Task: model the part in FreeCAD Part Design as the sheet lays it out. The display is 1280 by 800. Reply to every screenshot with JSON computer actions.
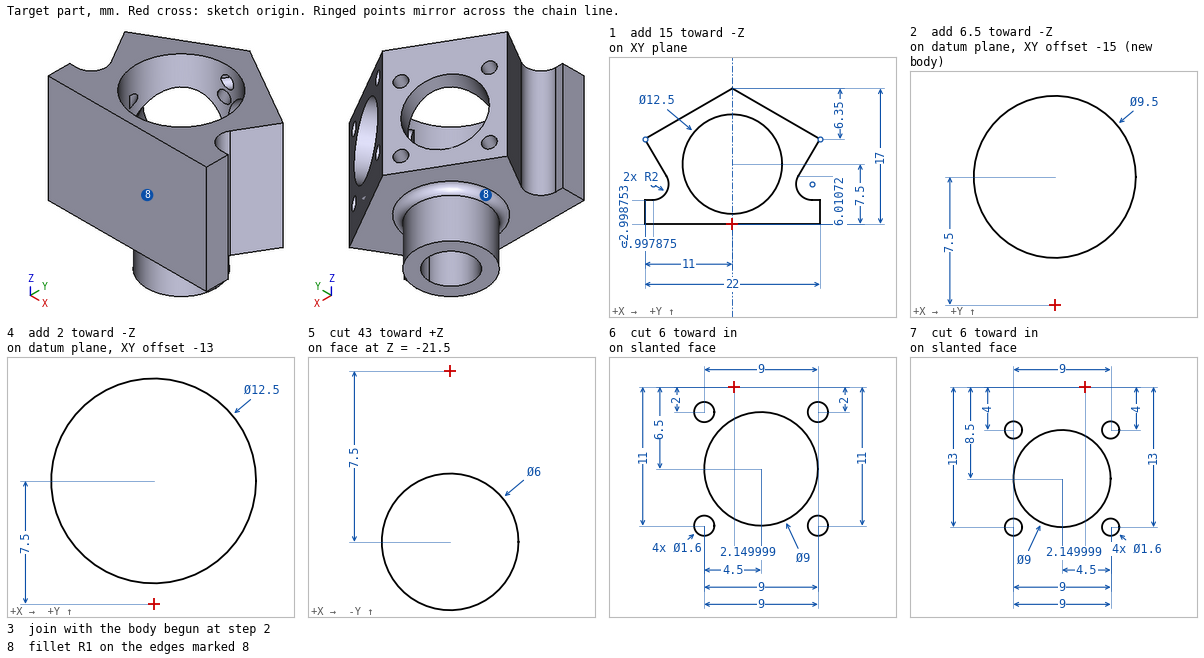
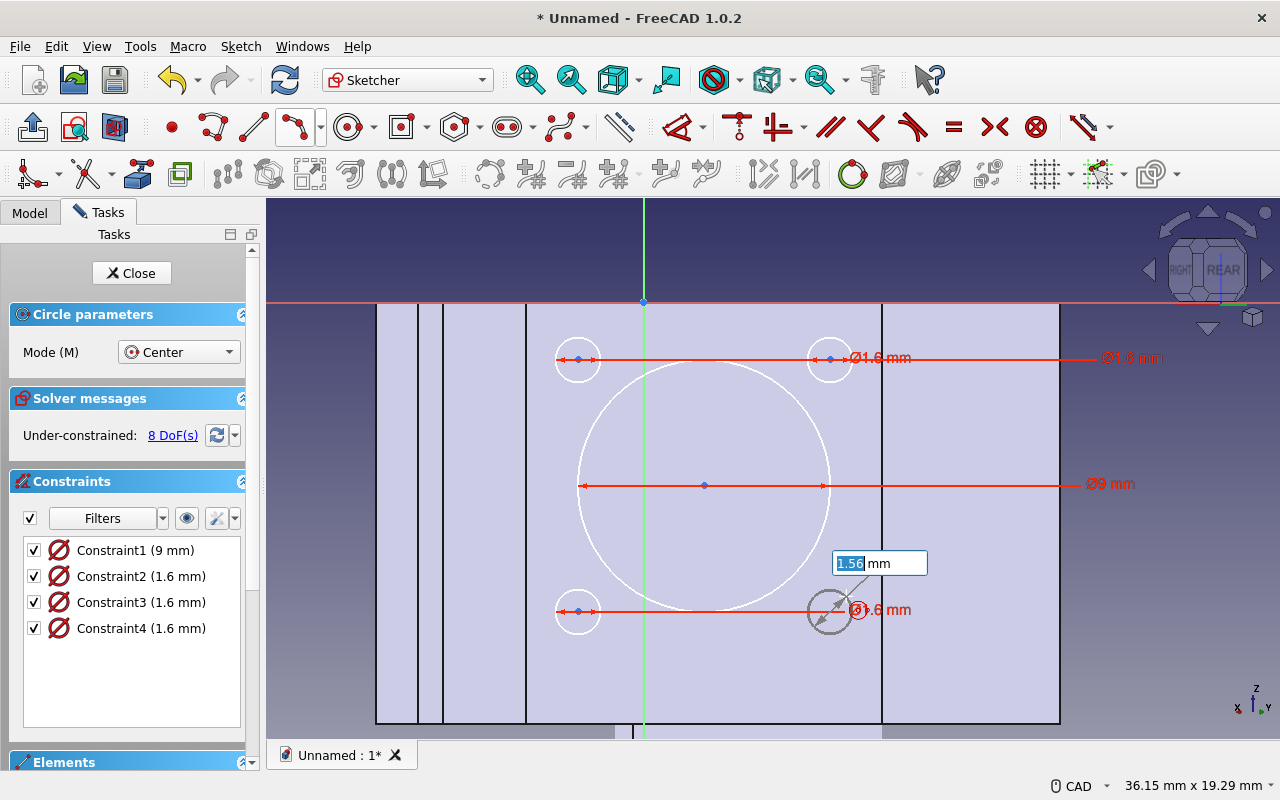
{"action": "type", "text": "1.6"}
{"action": "key", "text": "Return"}
{"action": "key", "text": "Escape"}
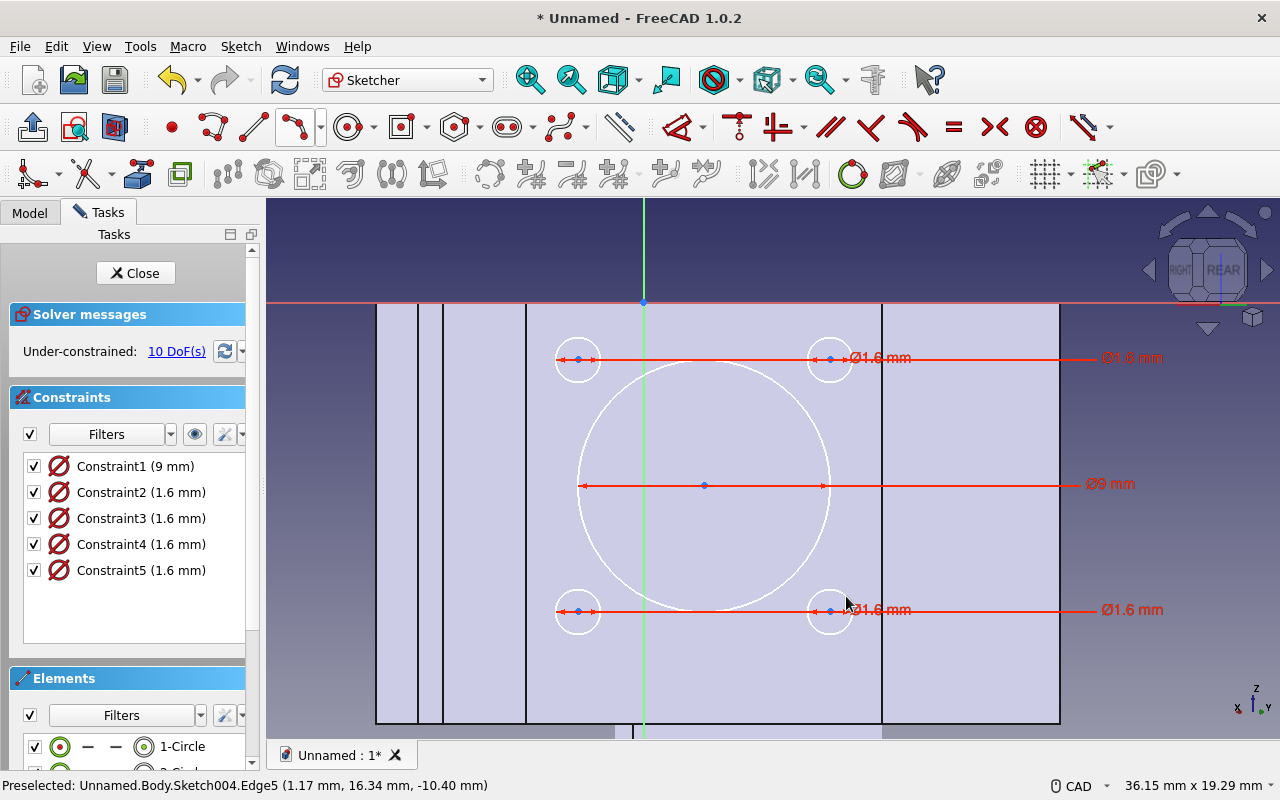
{"action": "left_click", "coordinate": [676, 128]}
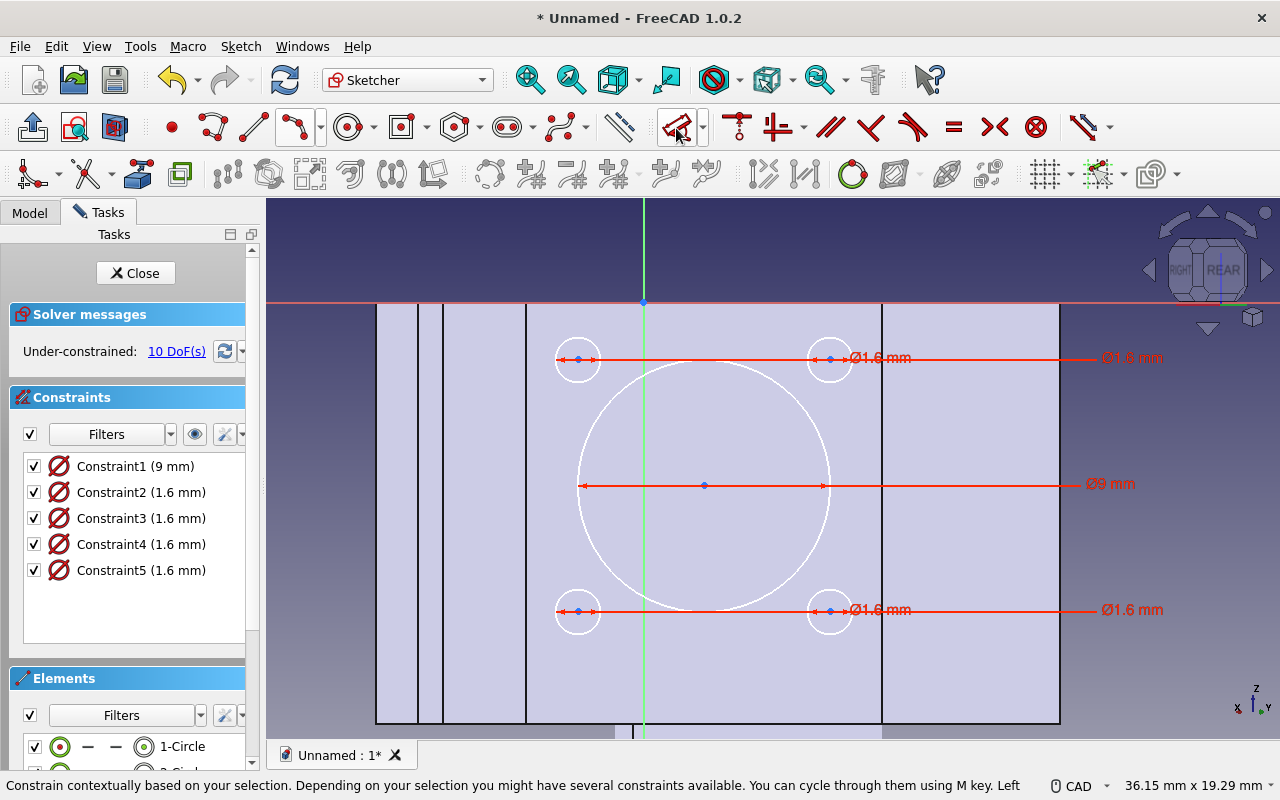
{"action": "left_click", "coordinate": [578, 360]}
{"action": "left_click", "coordinate": [544, 331]}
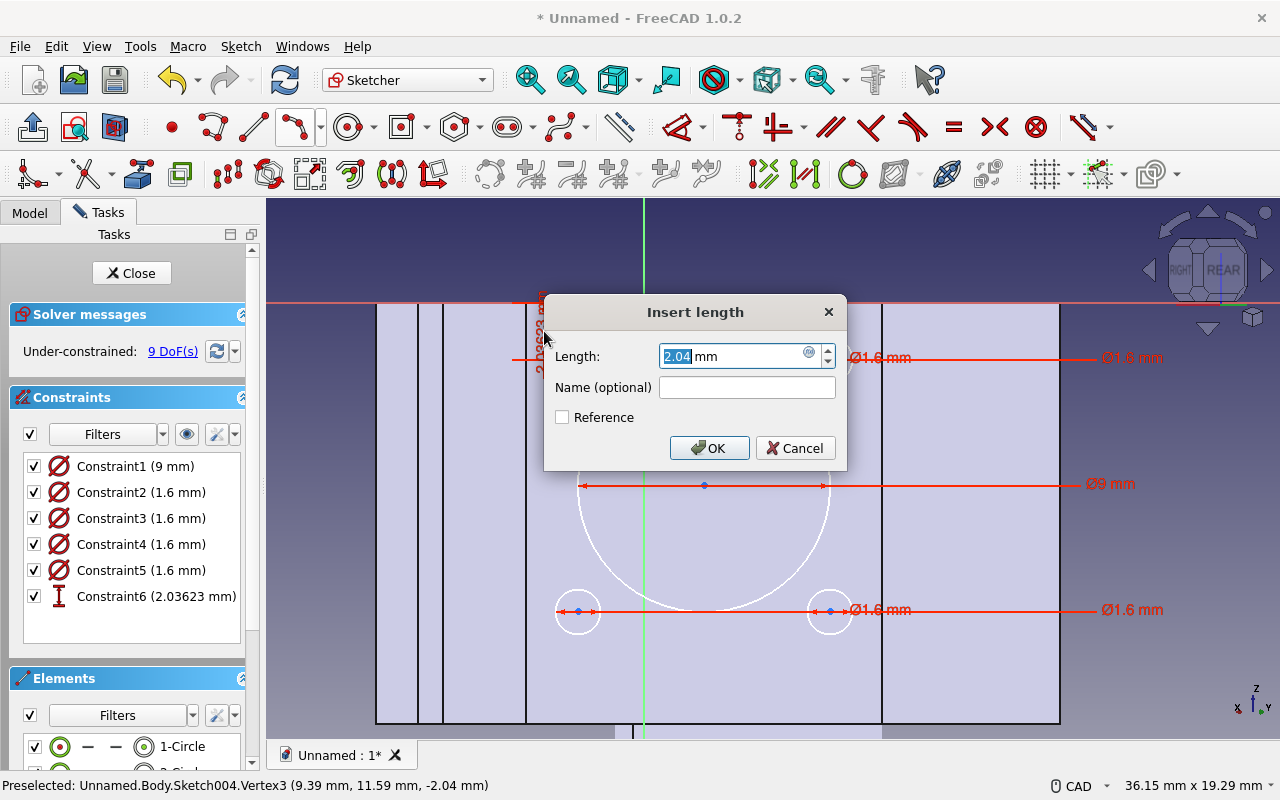
{"action": "type", "text": "2"}
{"action": "key", "text": "Return"}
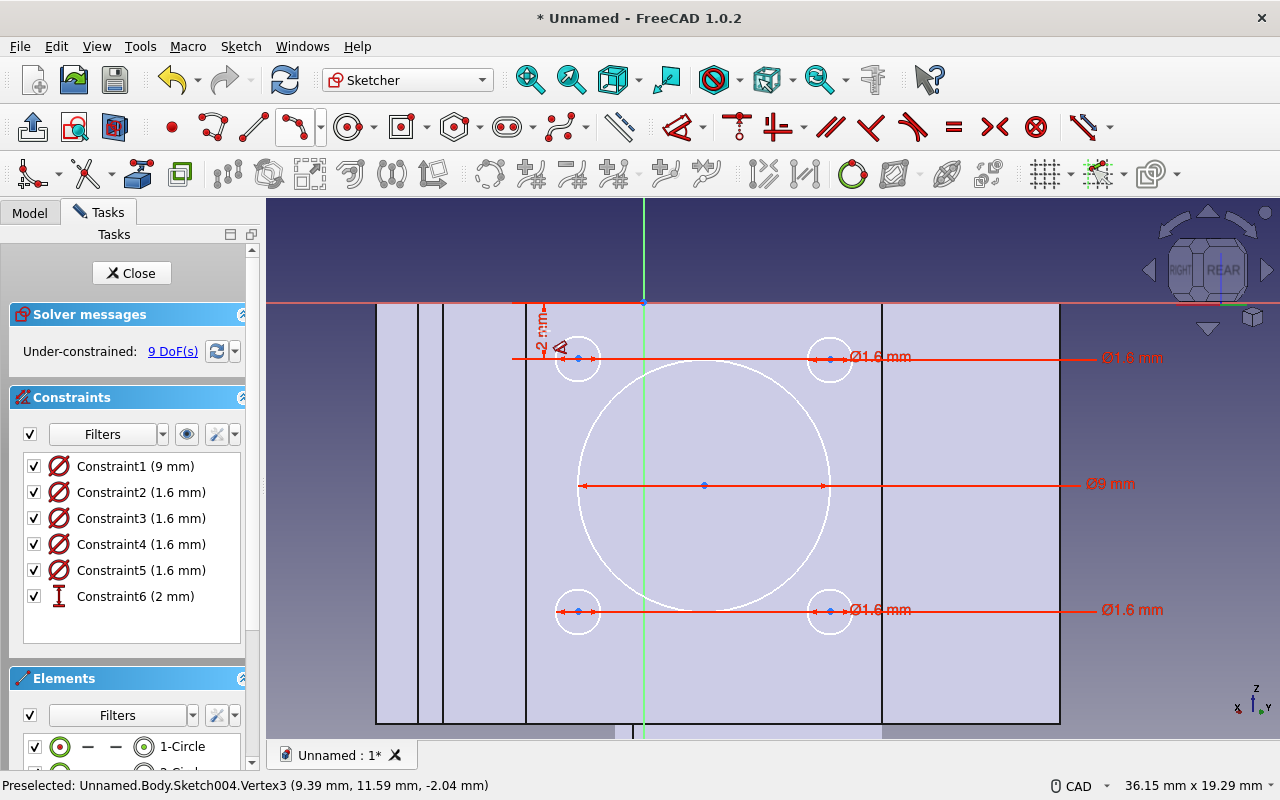
{"action": "left_click", "coordinate": [830, 360]}
{"action": "left_click", "coordinate": [864, 331]}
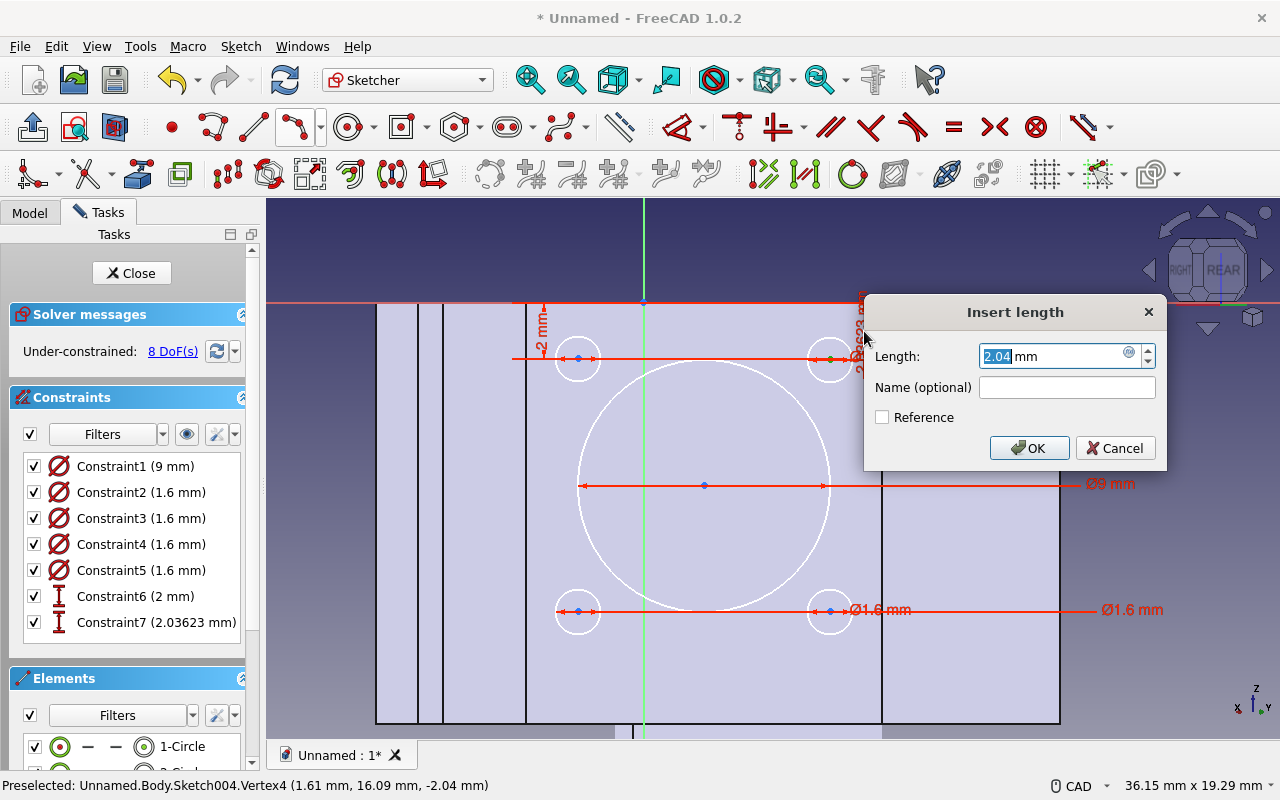
{"action": "type", "text": "2"}
{"action": "key", "text": "Return"}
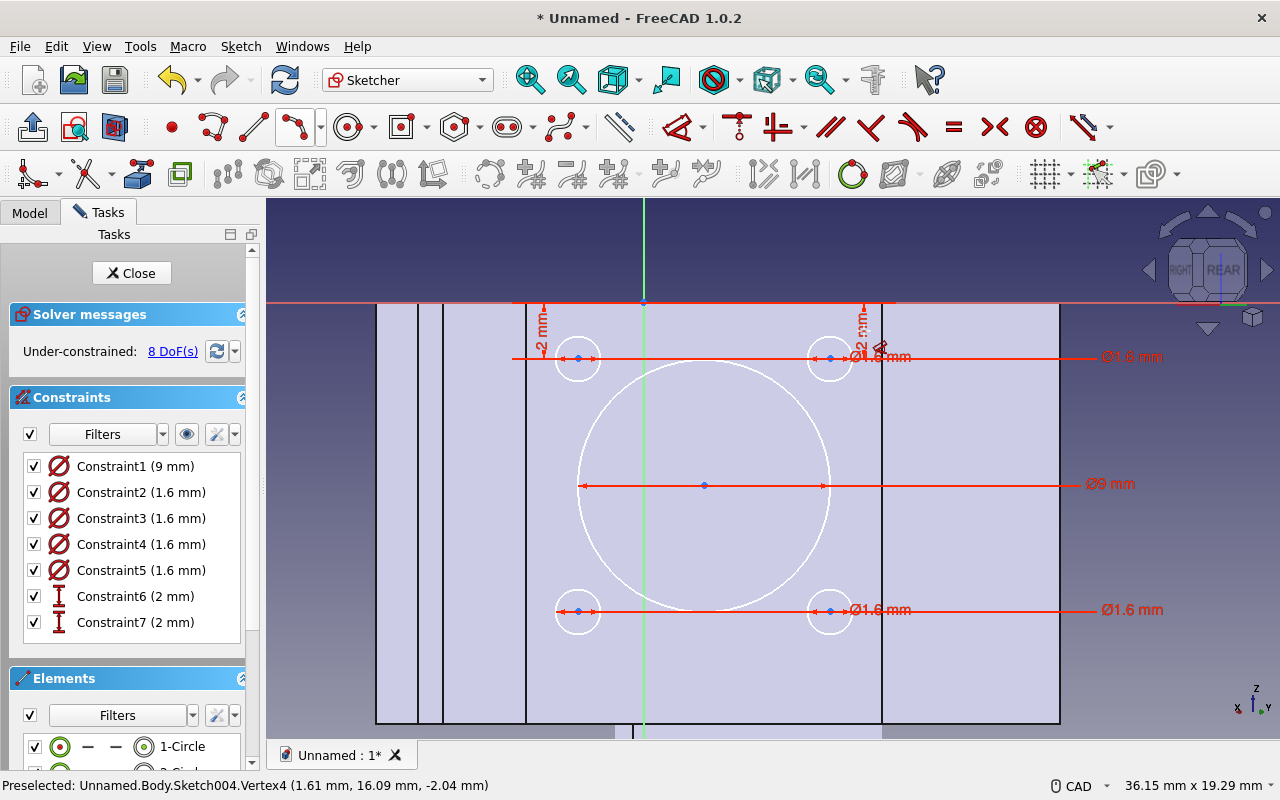
{"action": "left_click", "coordinate": [578, 612]}
{"action": "left_click", "coordinate": [544, 457]}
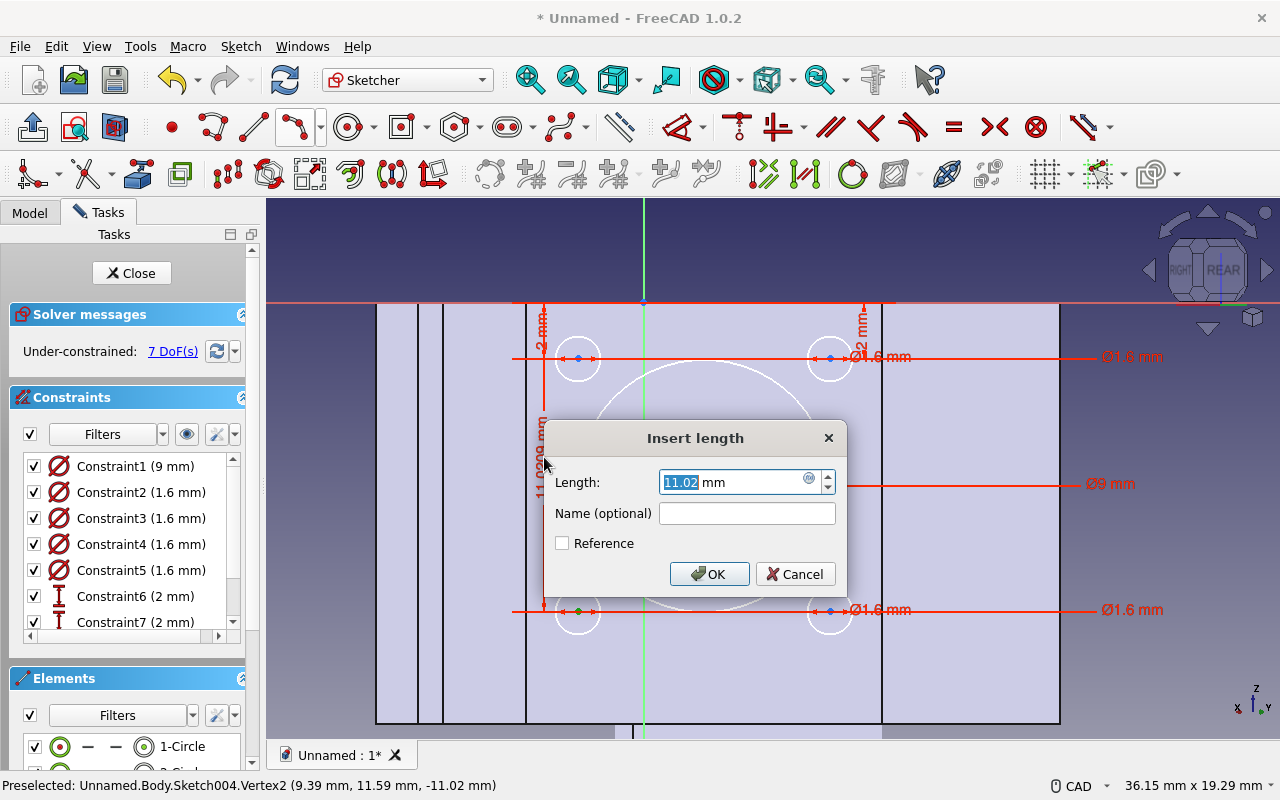
{"action": "type", "text": "11"}
{"action": "key", "text": "Return"}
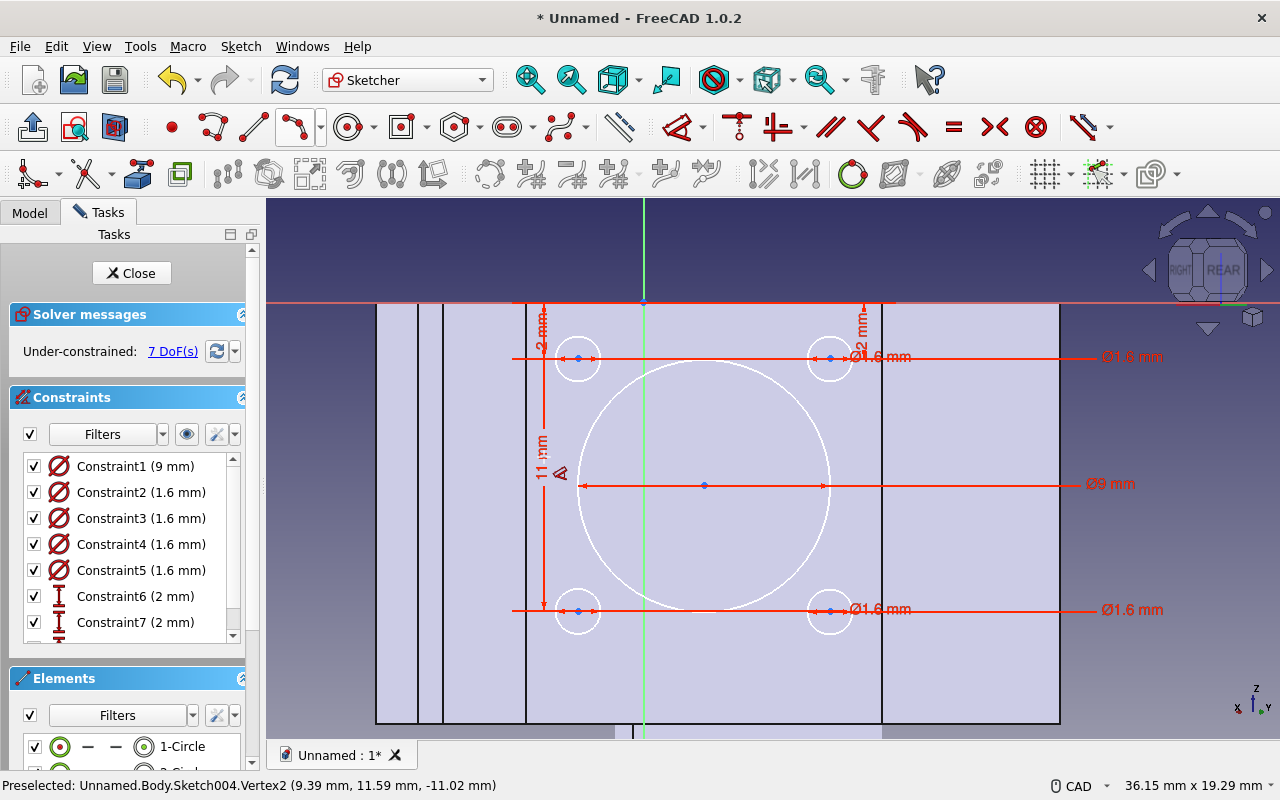
{"action": "left_click", "coordinate": [830, 612]}
{"action": "left_click", "coordinate": [864, 457]}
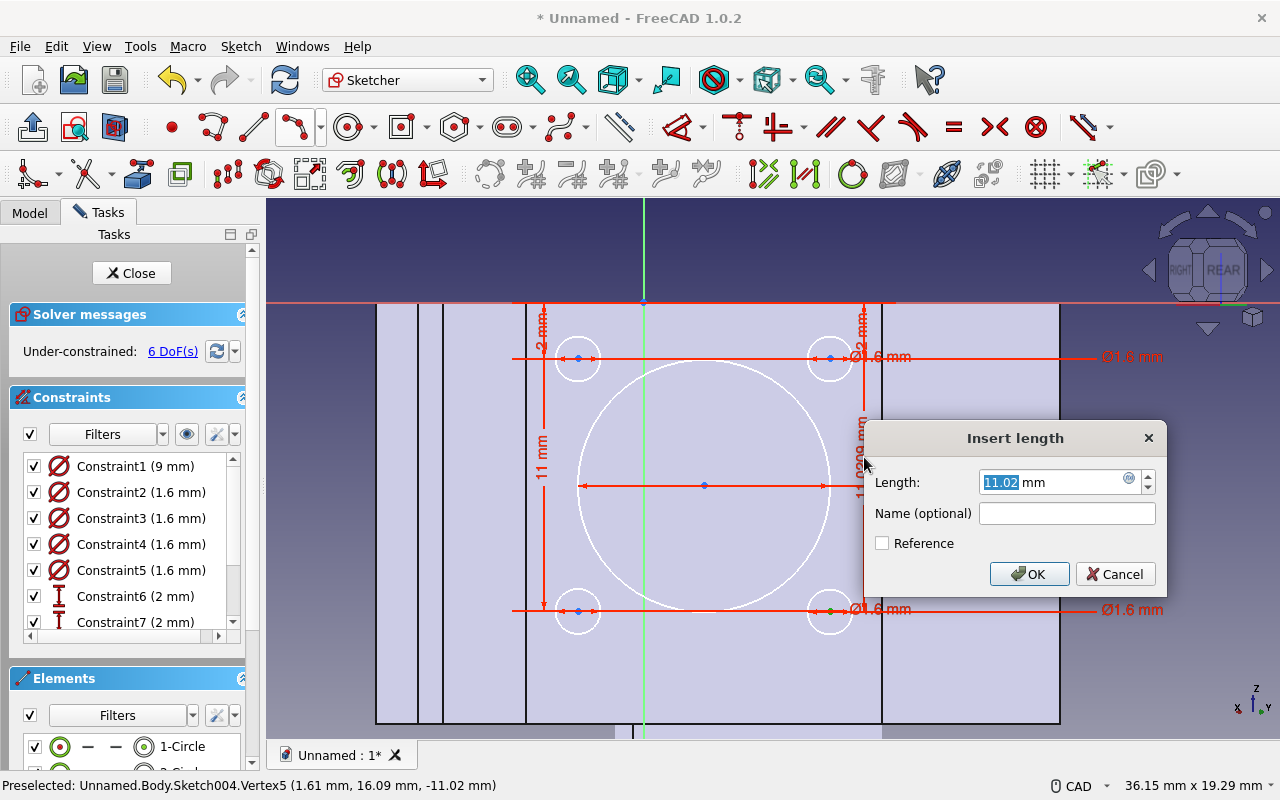
{"action": "type", "text": "11"}
{"action": "key", "text": "Return"}